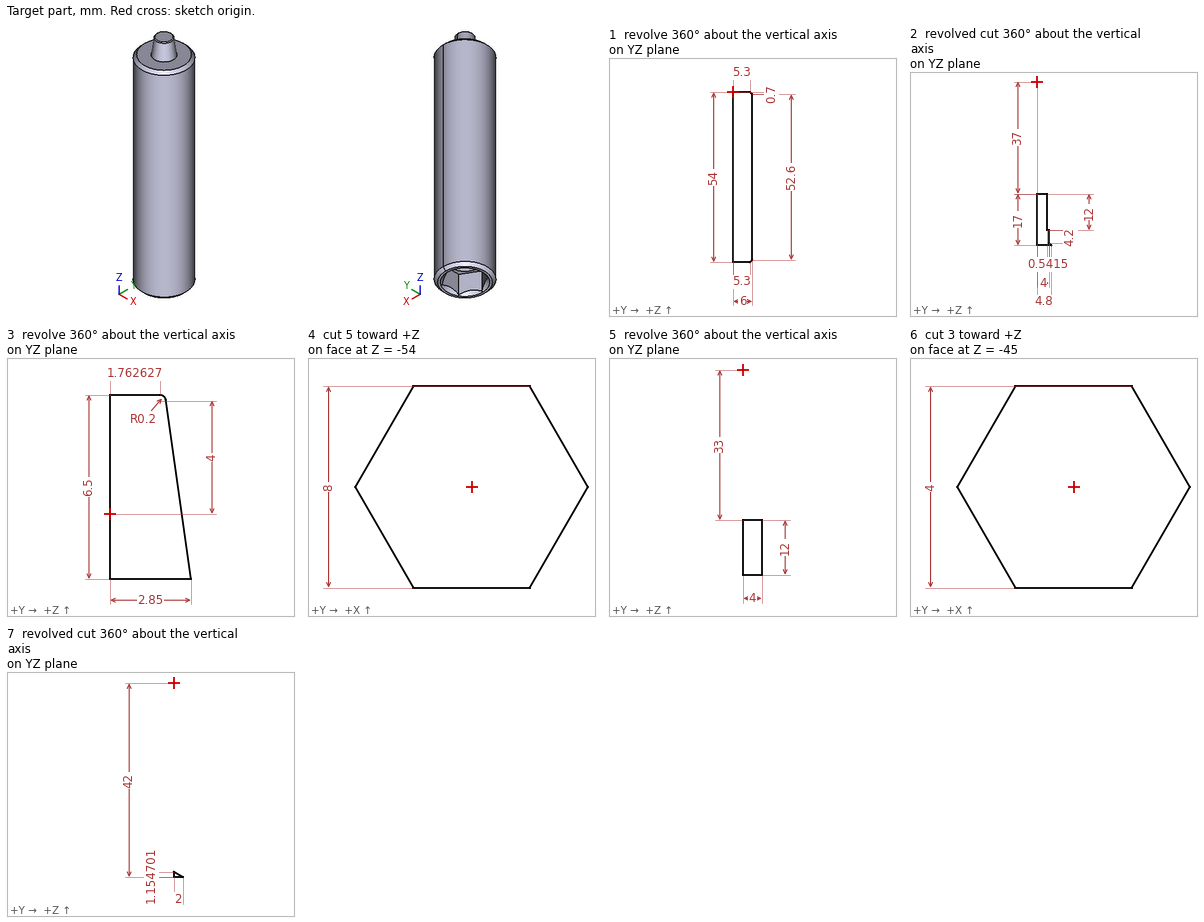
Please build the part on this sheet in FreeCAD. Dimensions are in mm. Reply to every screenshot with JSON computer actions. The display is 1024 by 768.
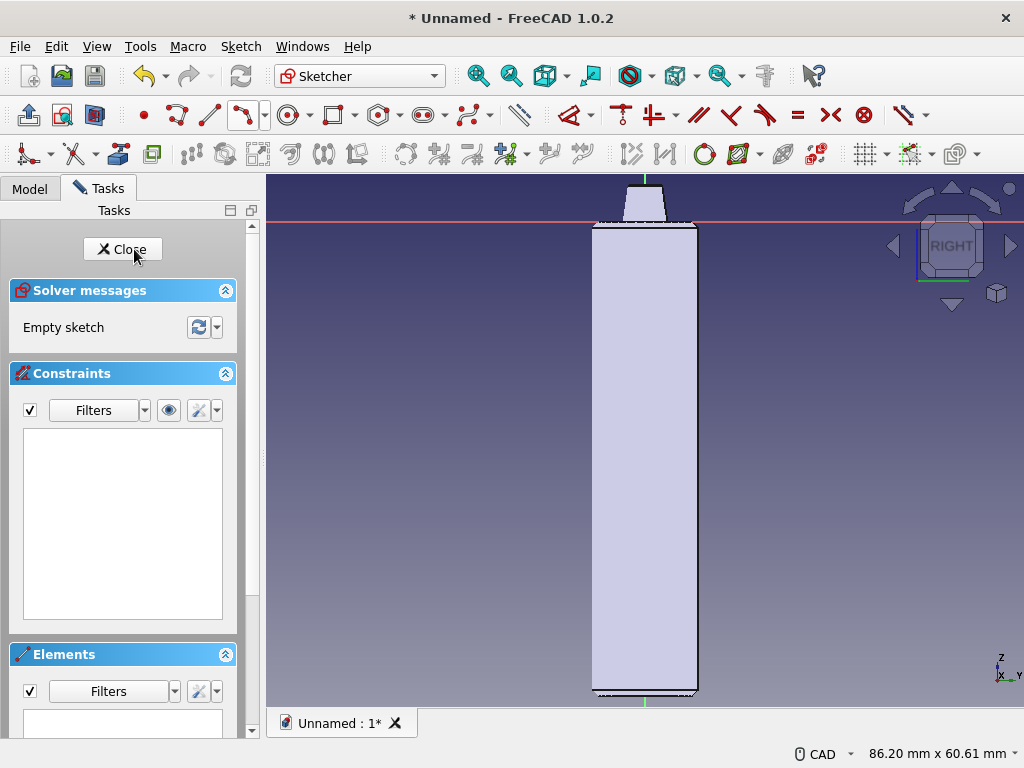
{"action": "left_click", "coordinate": [95, 116]}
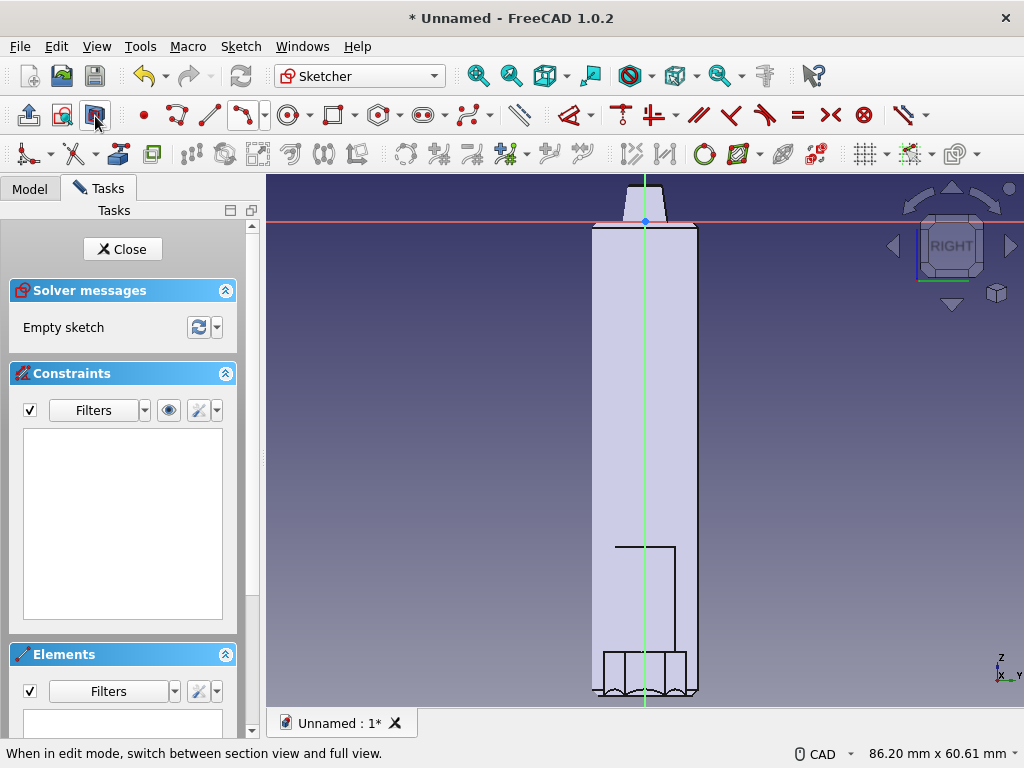
{"action": "scroll", "coordinate": [700, 618], "scroll_direction": "up", "scroll_amount": 6}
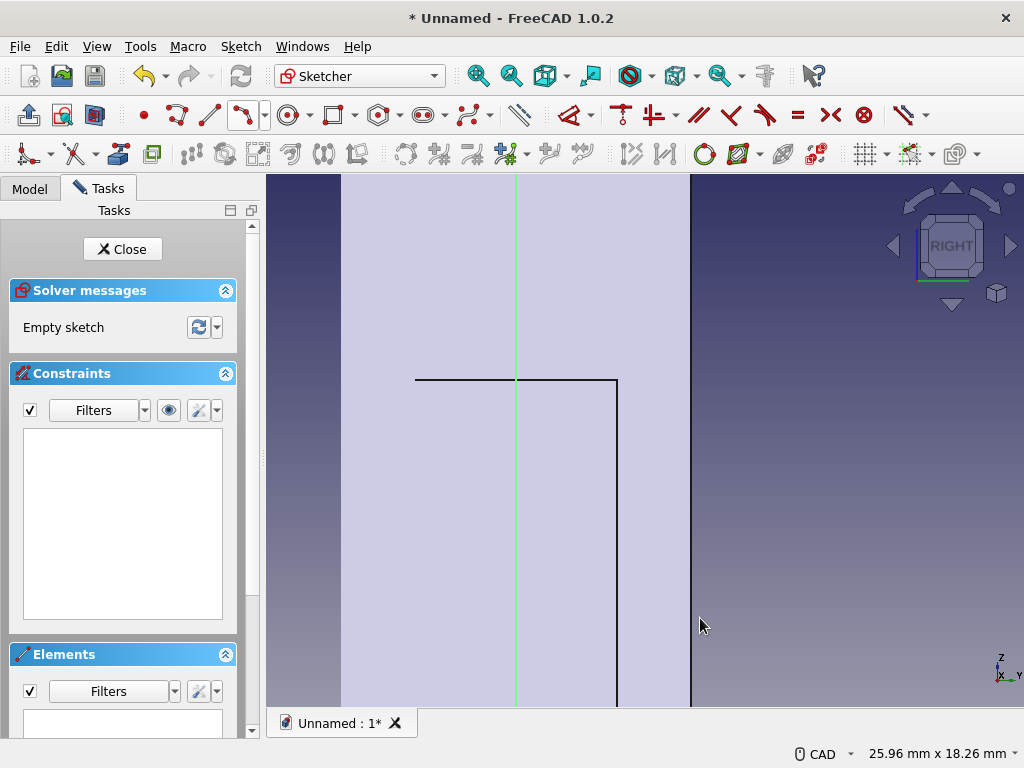
{"action": "left_click", "coordinate": [332, 116]}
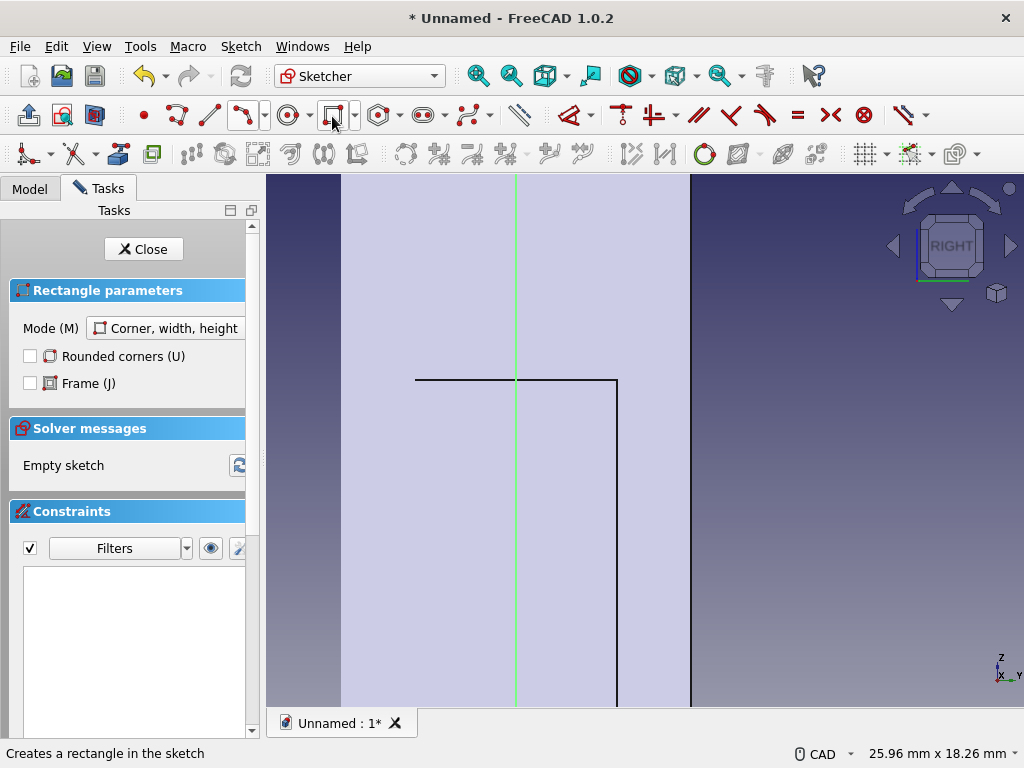
{"action": "left_click", "coordinate": [516, 263]}
{"action": "mouse_move", "coordinate": [633, 614]}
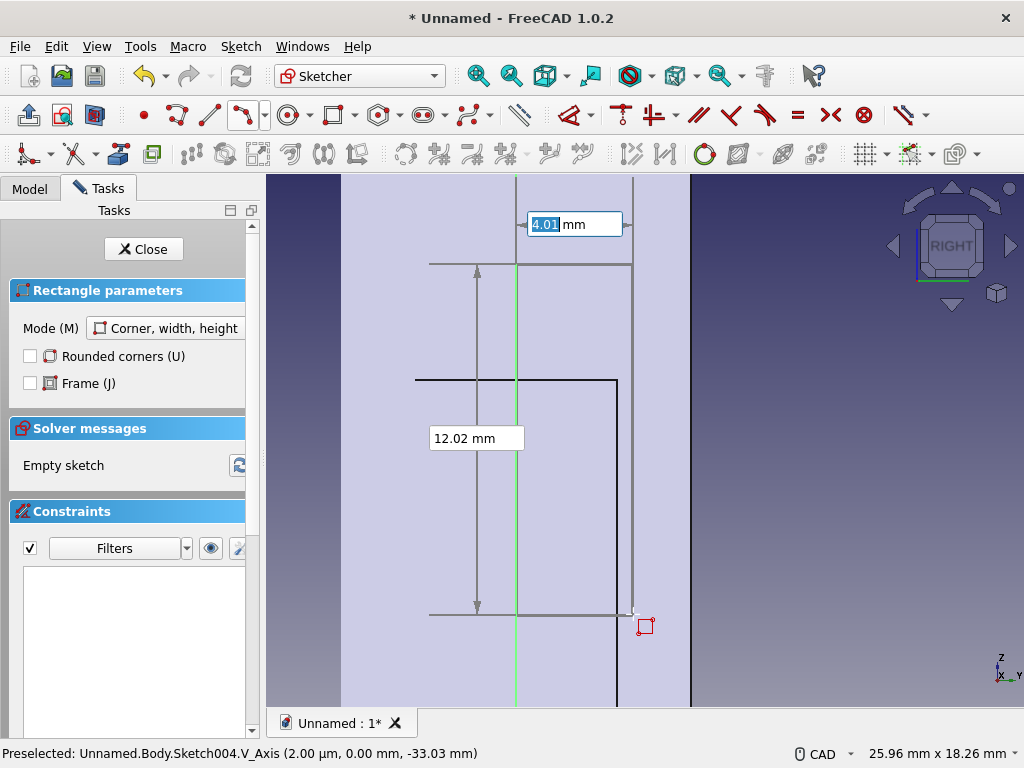
{"action": "type", "text": "4"}
{"action": "key", "text": "Tab"}
{"action": "type", "text": "12"}
{"action": "key", "text": "Return"}
{"action": "key", "text": "Escape"}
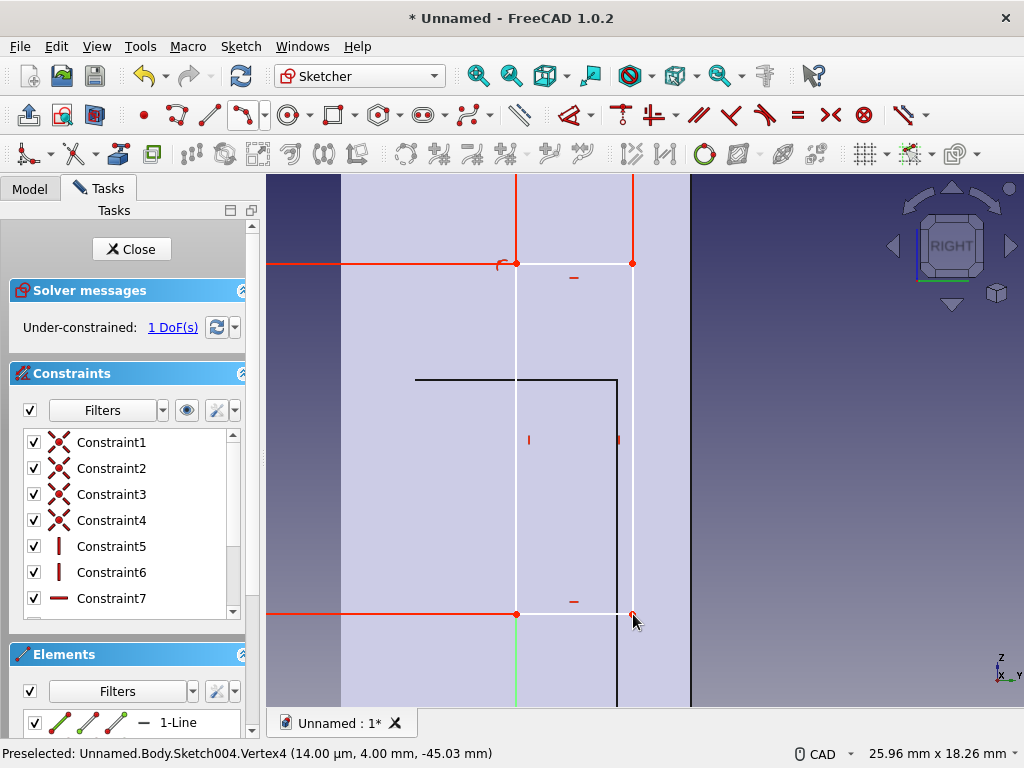
{"action": "left_click", "coordinate": [568, 116]}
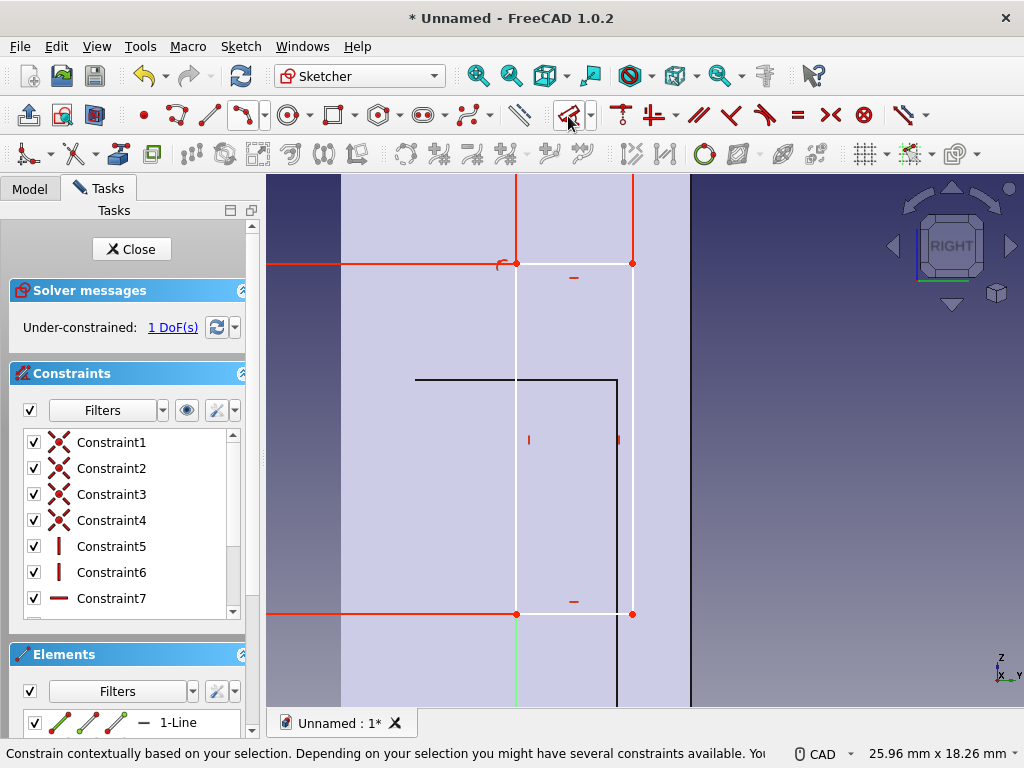
{"action": "left_click", "coordinate": [516, 264]}
{"action": "left_click", "coordinate": [482, 233]}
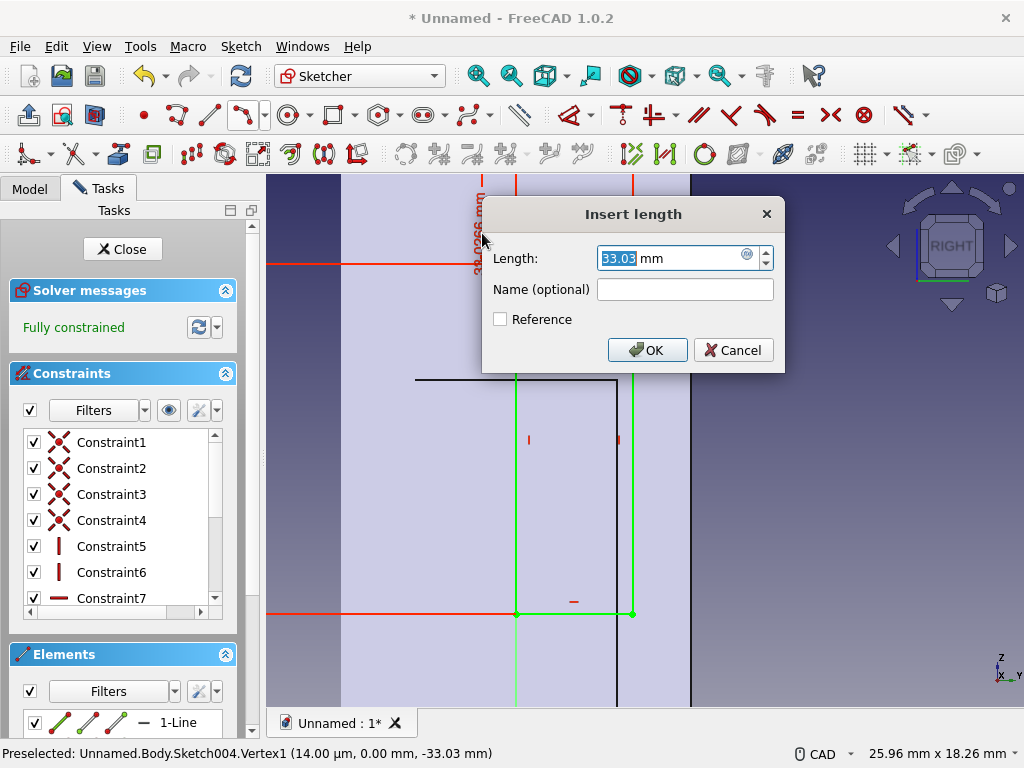
{"action": "type", "text": "33"}
{"action": "key", "text": "Return"}
{"action": "key", "text": "Escape"}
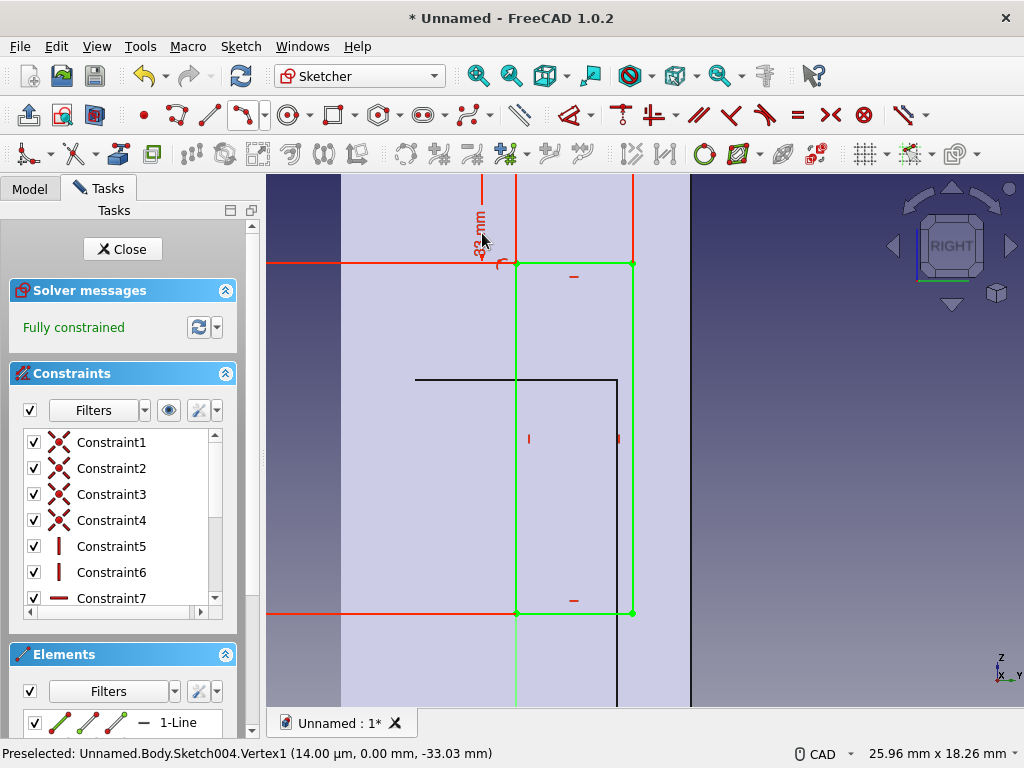
{"action": "left_click", "coordinate": [123, 249]}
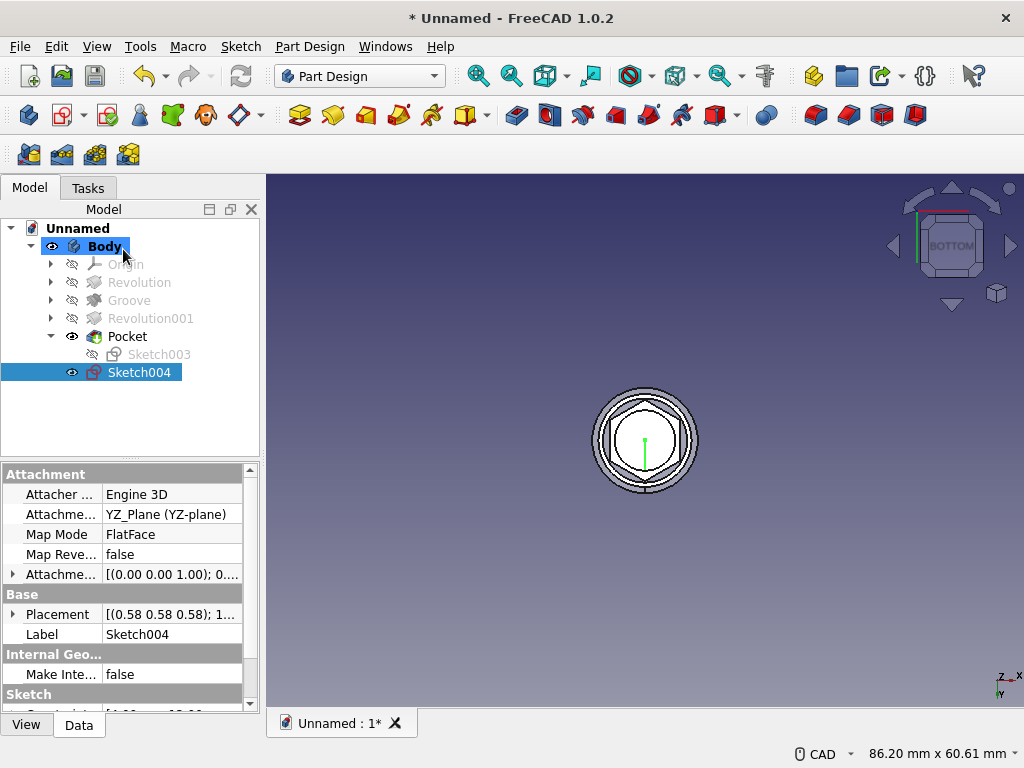
{"action": "left_click", "coordinate": [333, 116]}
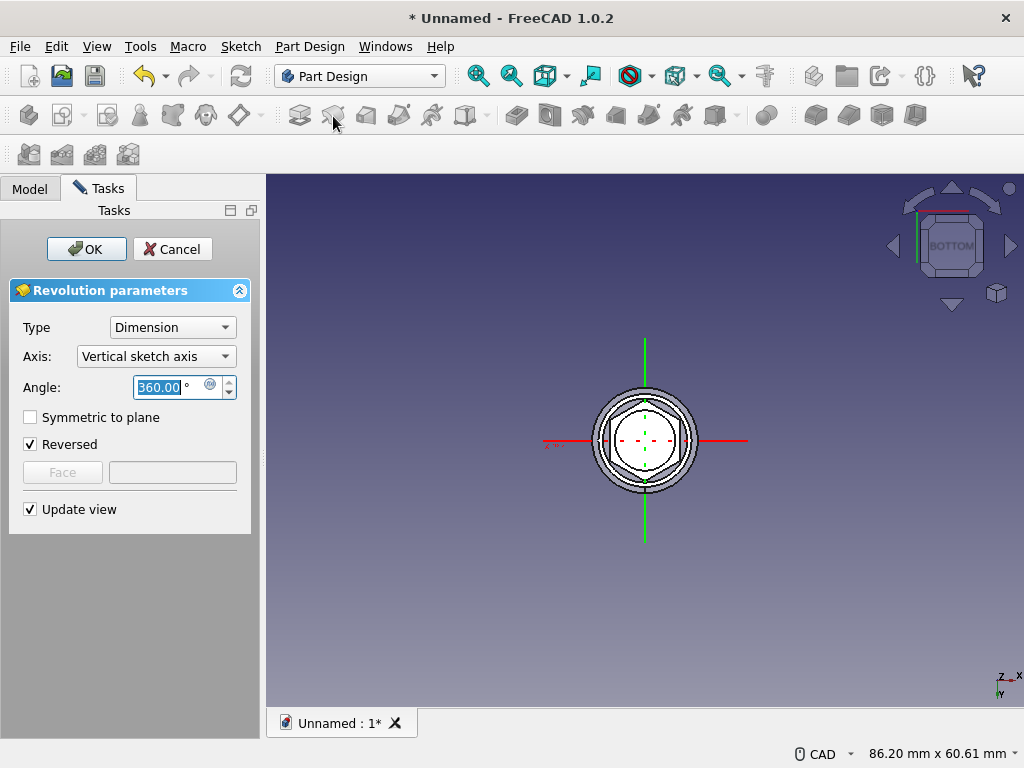
{"action": "left_click", "coordinate": [87, 249]}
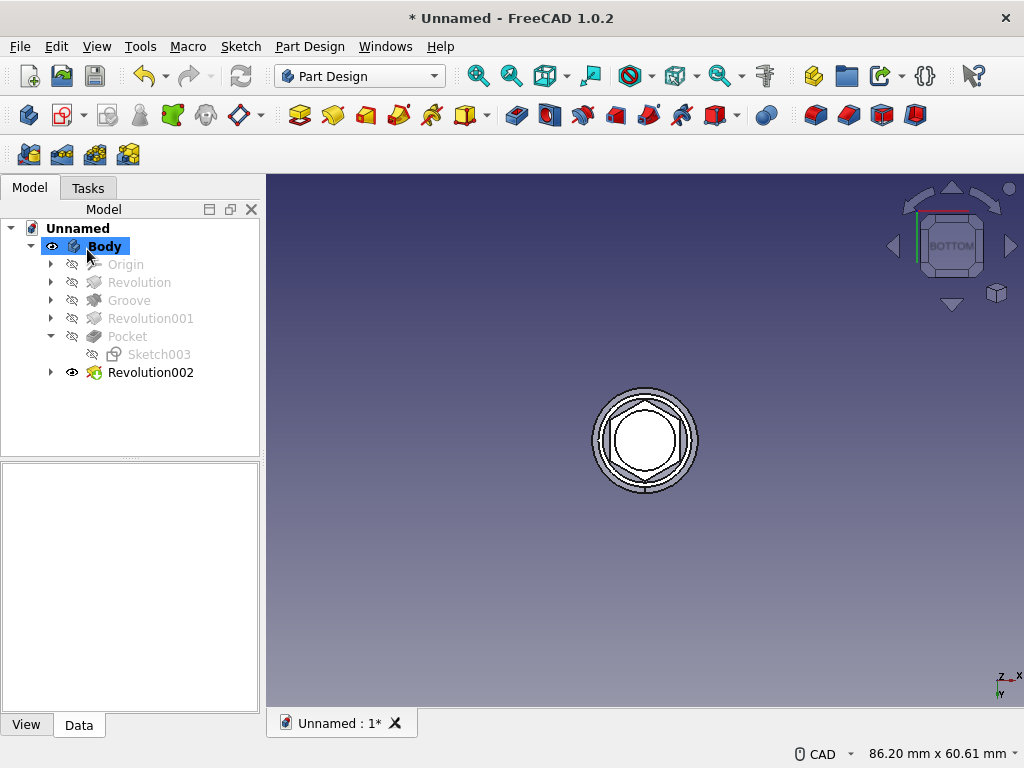
{"action": "left_click", "coordinate": [479, 76]}